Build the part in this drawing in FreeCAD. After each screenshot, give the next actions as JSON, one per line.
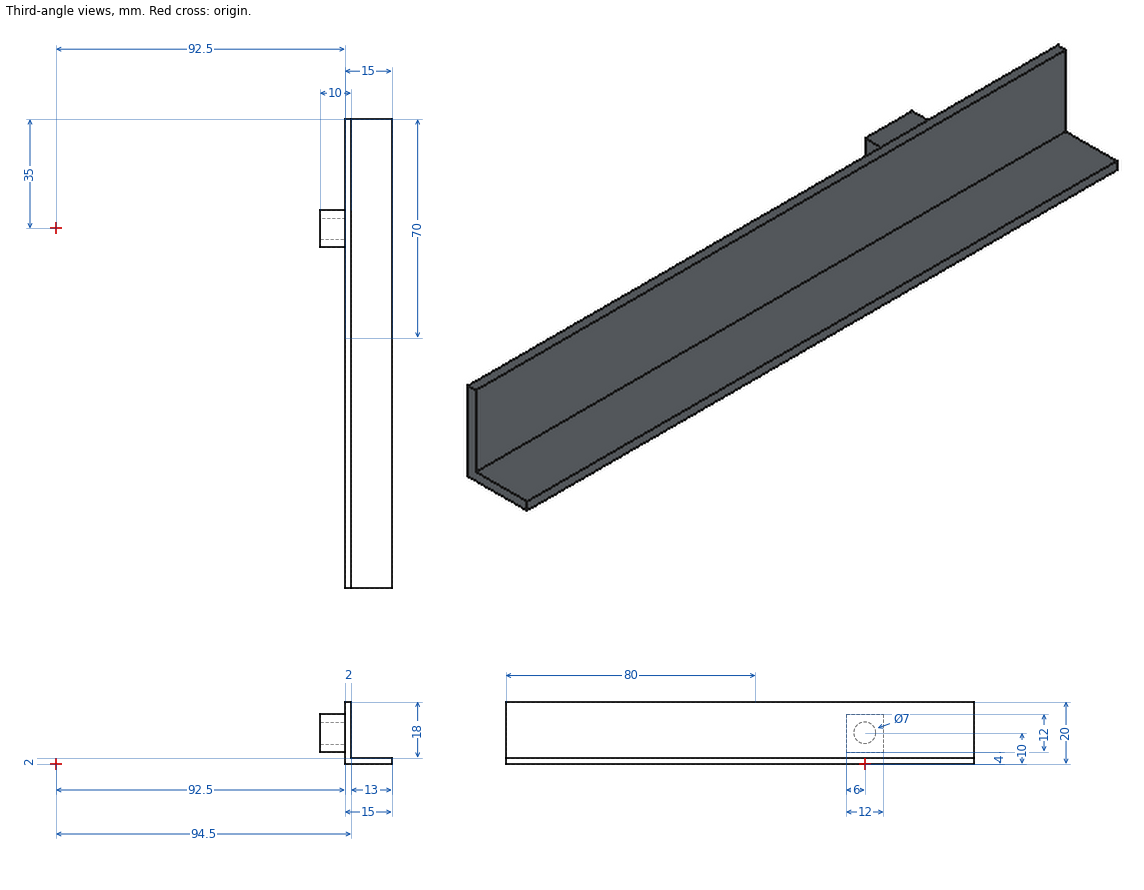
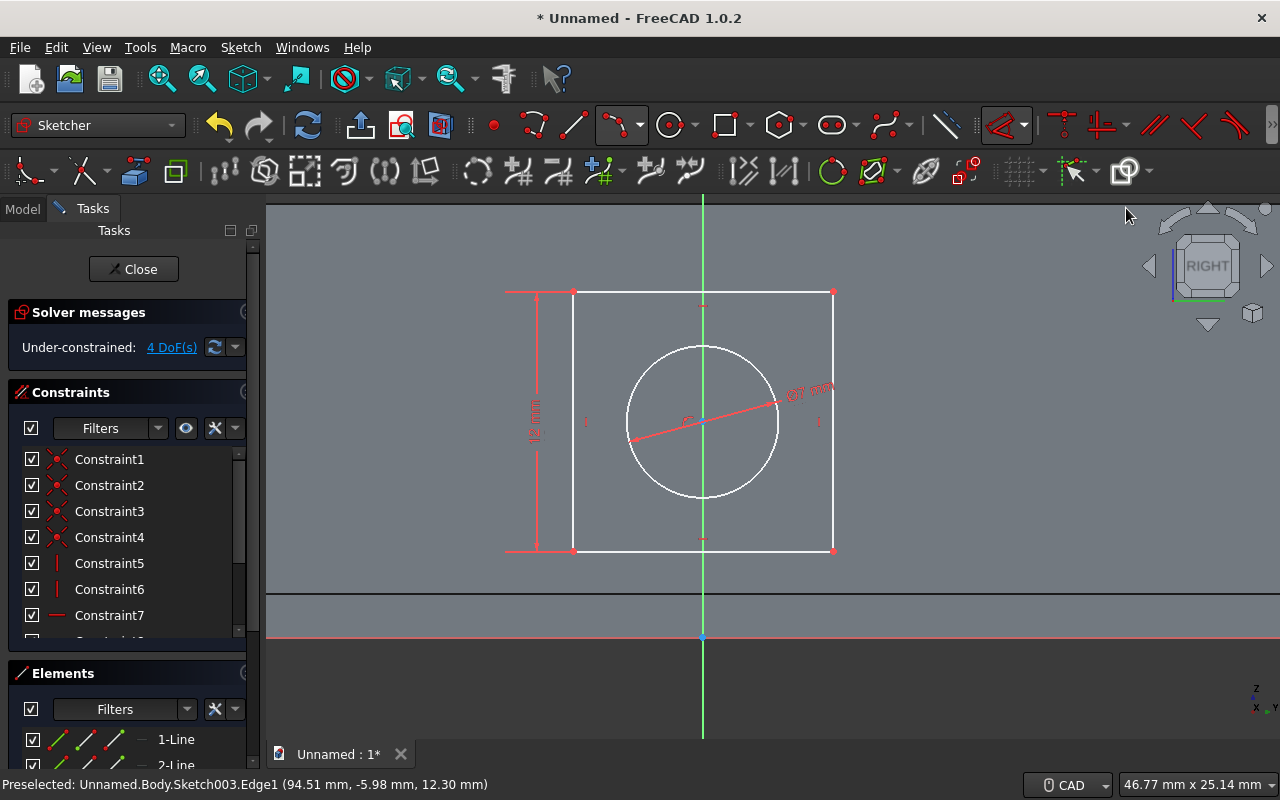
{"action": "left_click", "coordinate": [651, 552]}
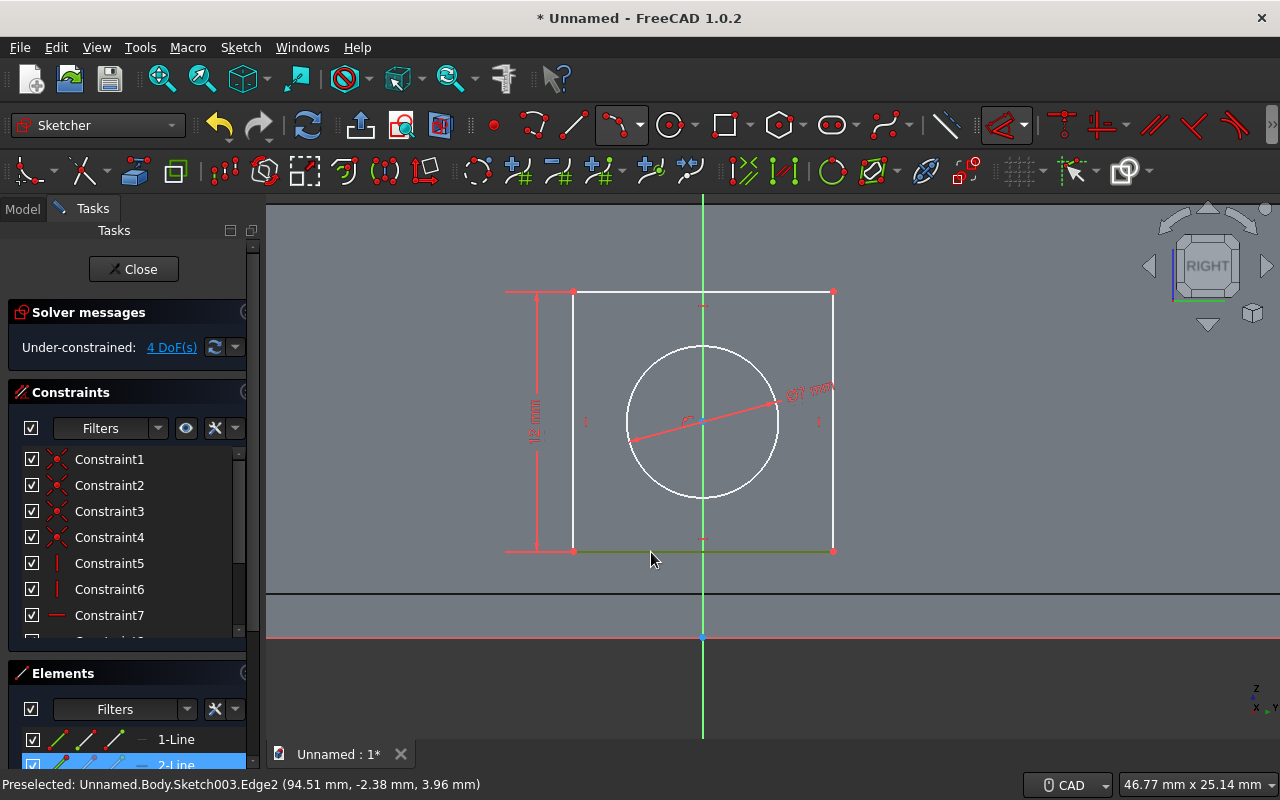
{"action": "key", "text": "l"}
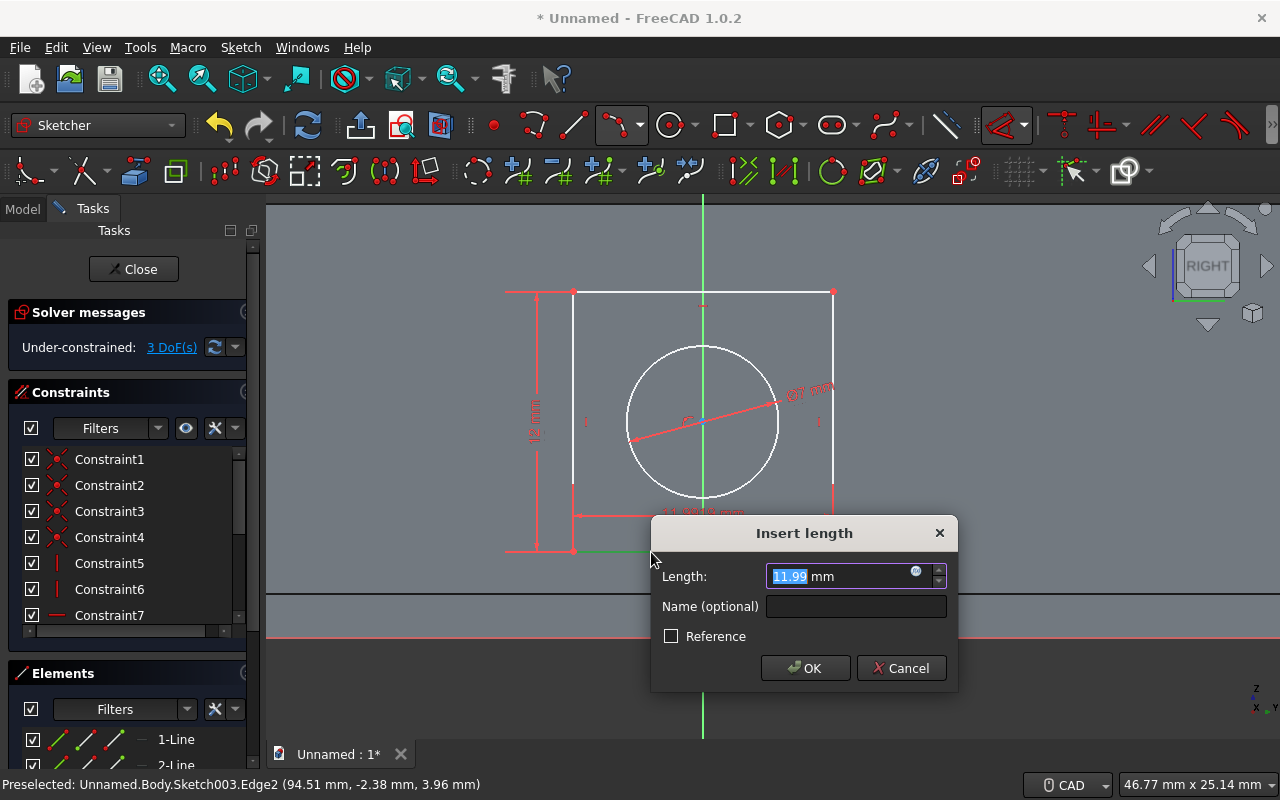
{"action": "type", "text": "12"}
{"action": "key", "text": "Return"}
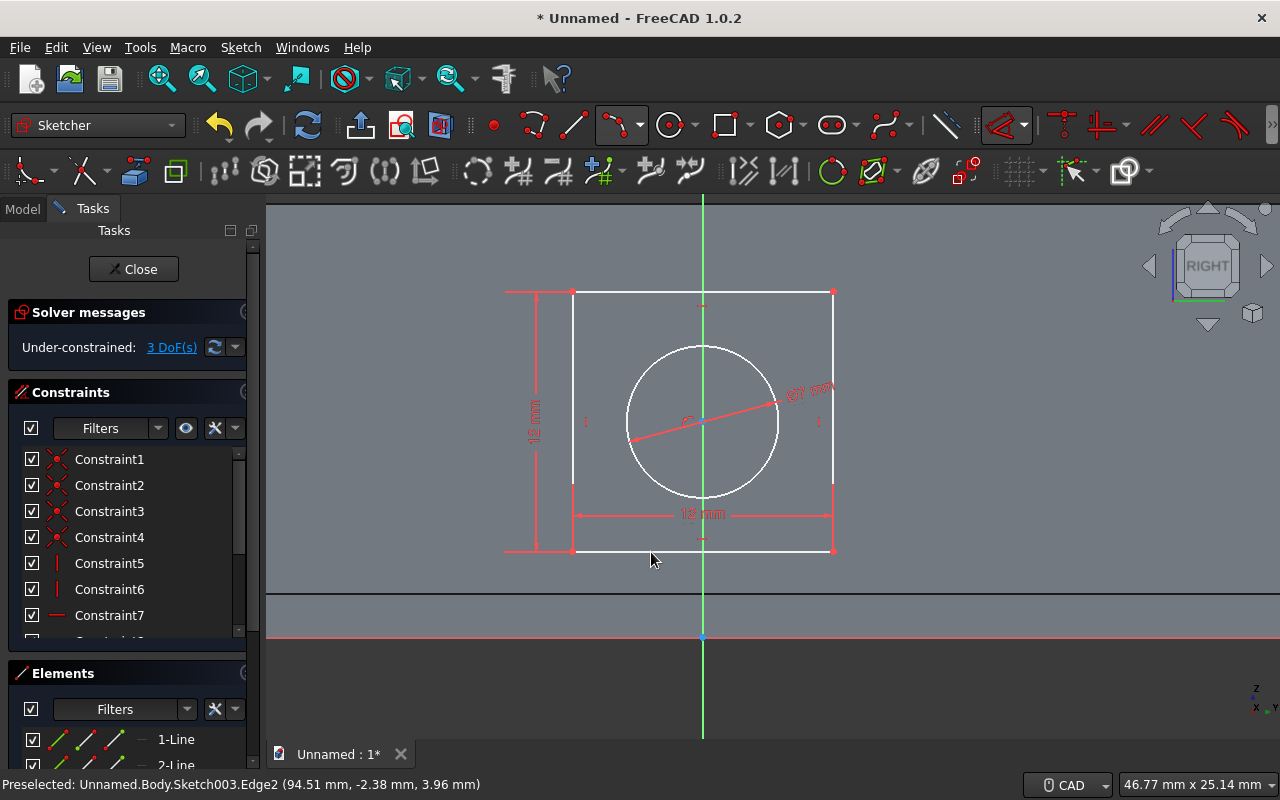
{"action": "left_click", "coordinate": [573, 292]}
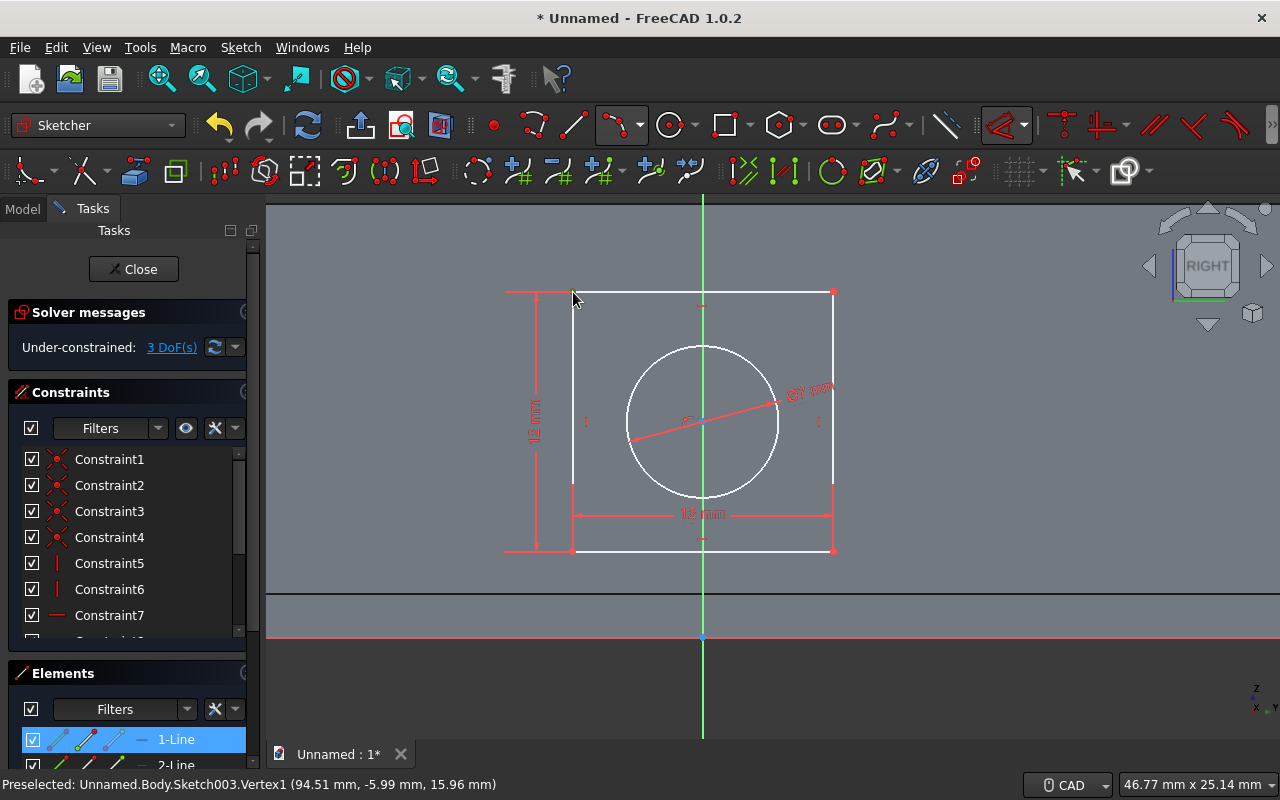
{"action": "left_click", "coordinate": [1026, 126]}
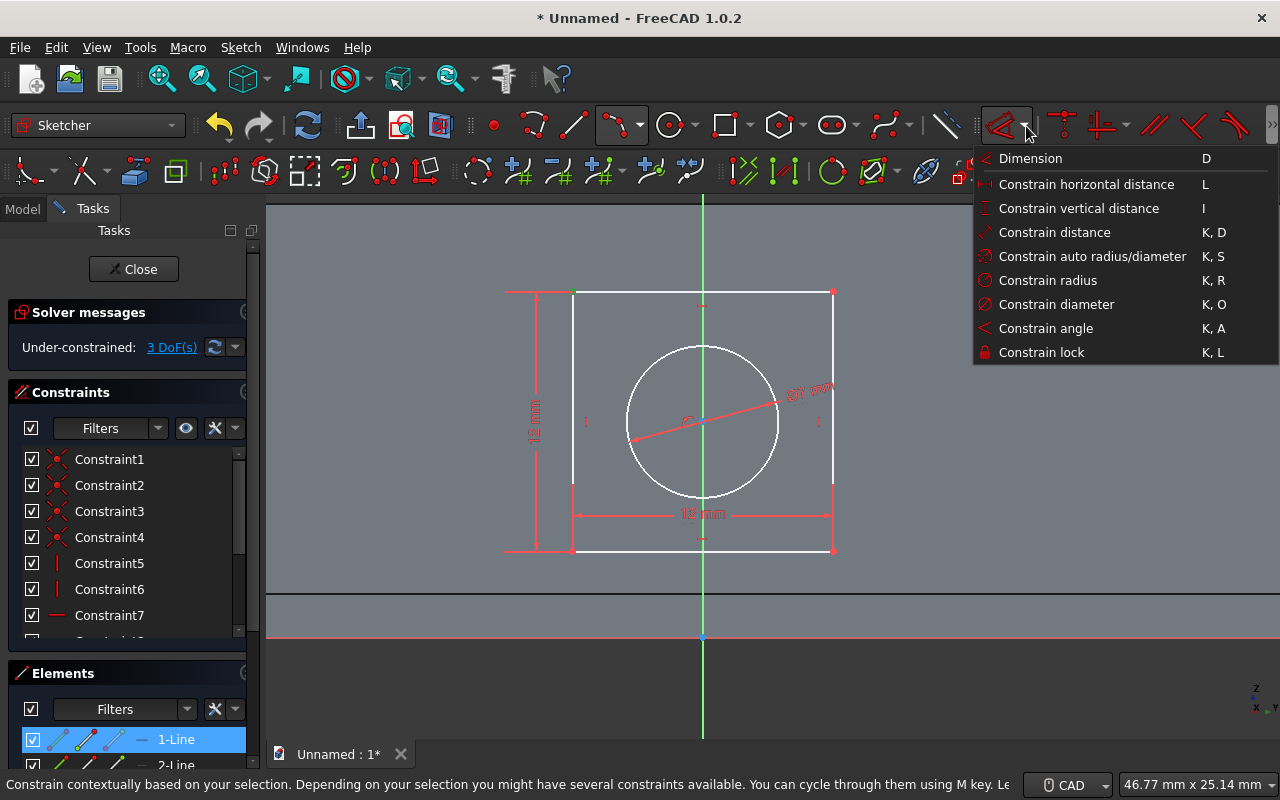
{"action": "left_click", "coordinate": [1126, 184]}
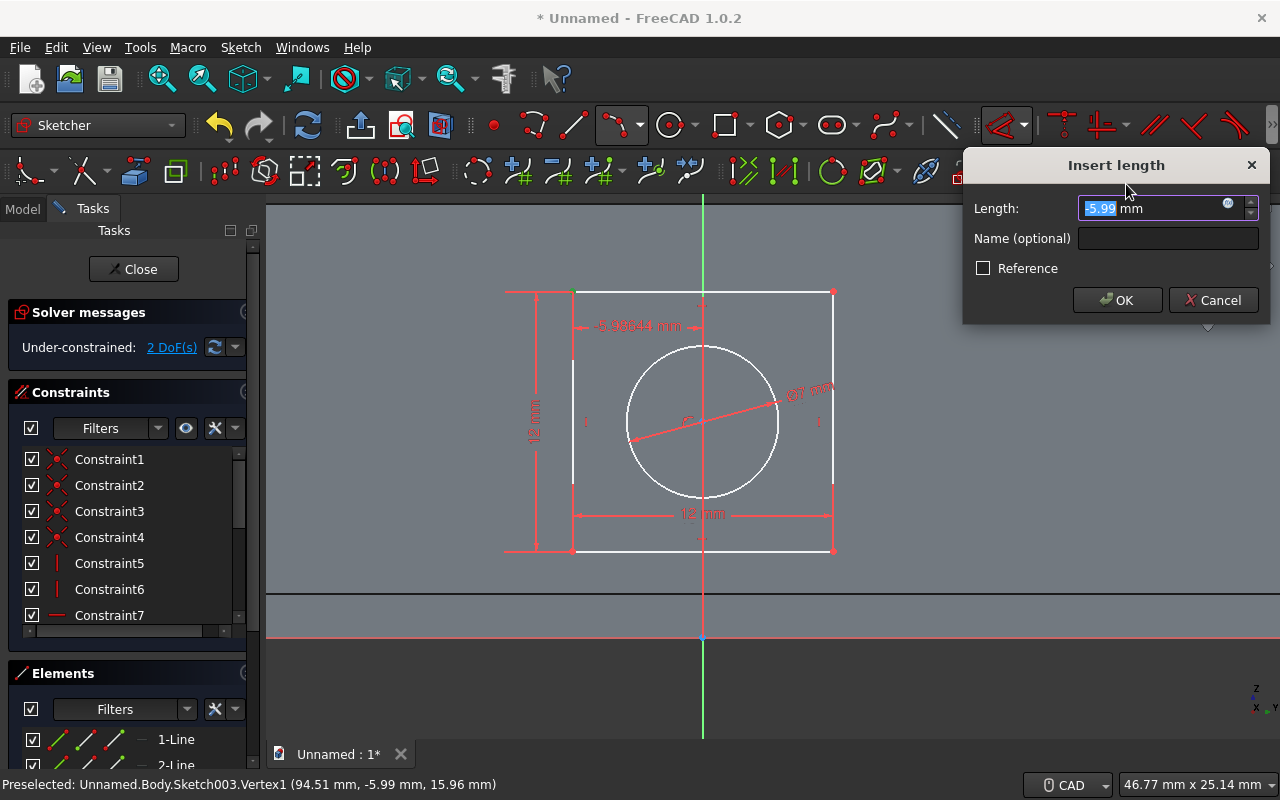
{"action": "type", "text": "-6"}
{"action": "key", "text": "Return"}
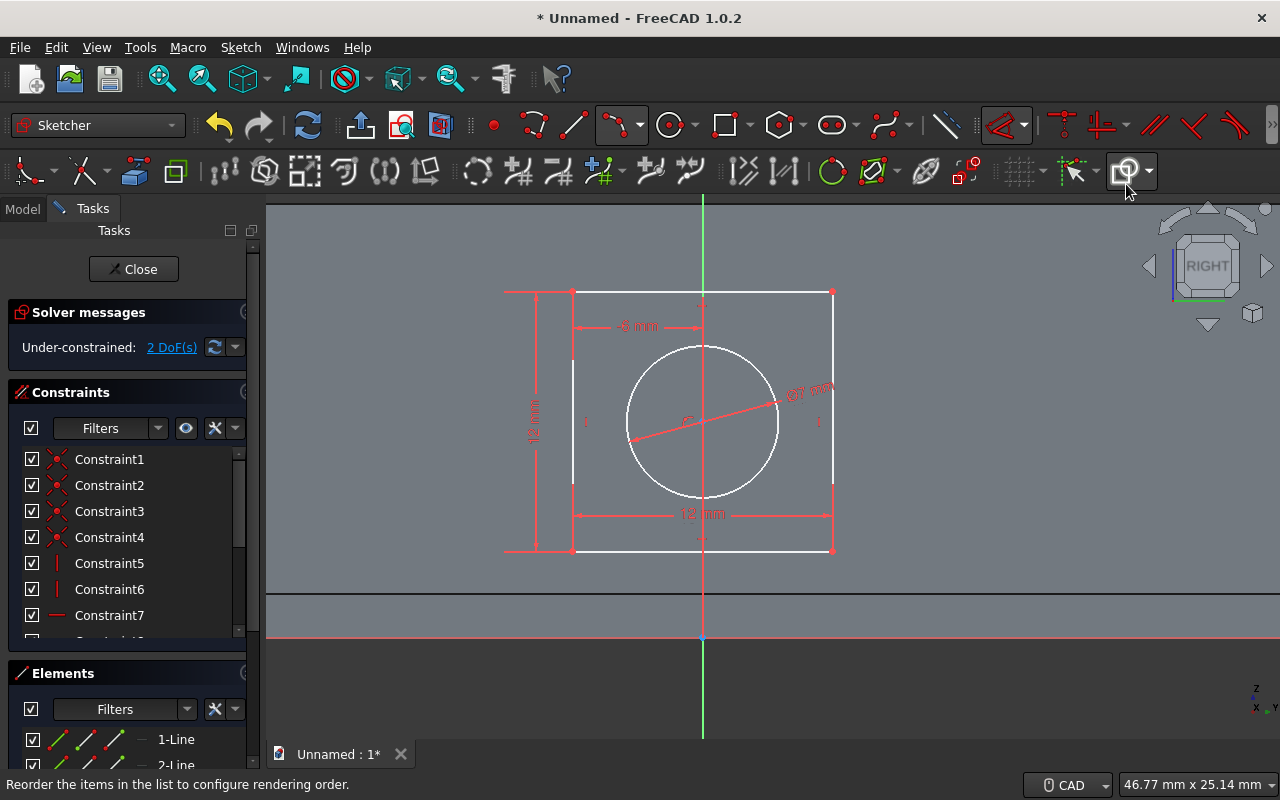
{"action": "left_click", "coordinate": [573, 552]}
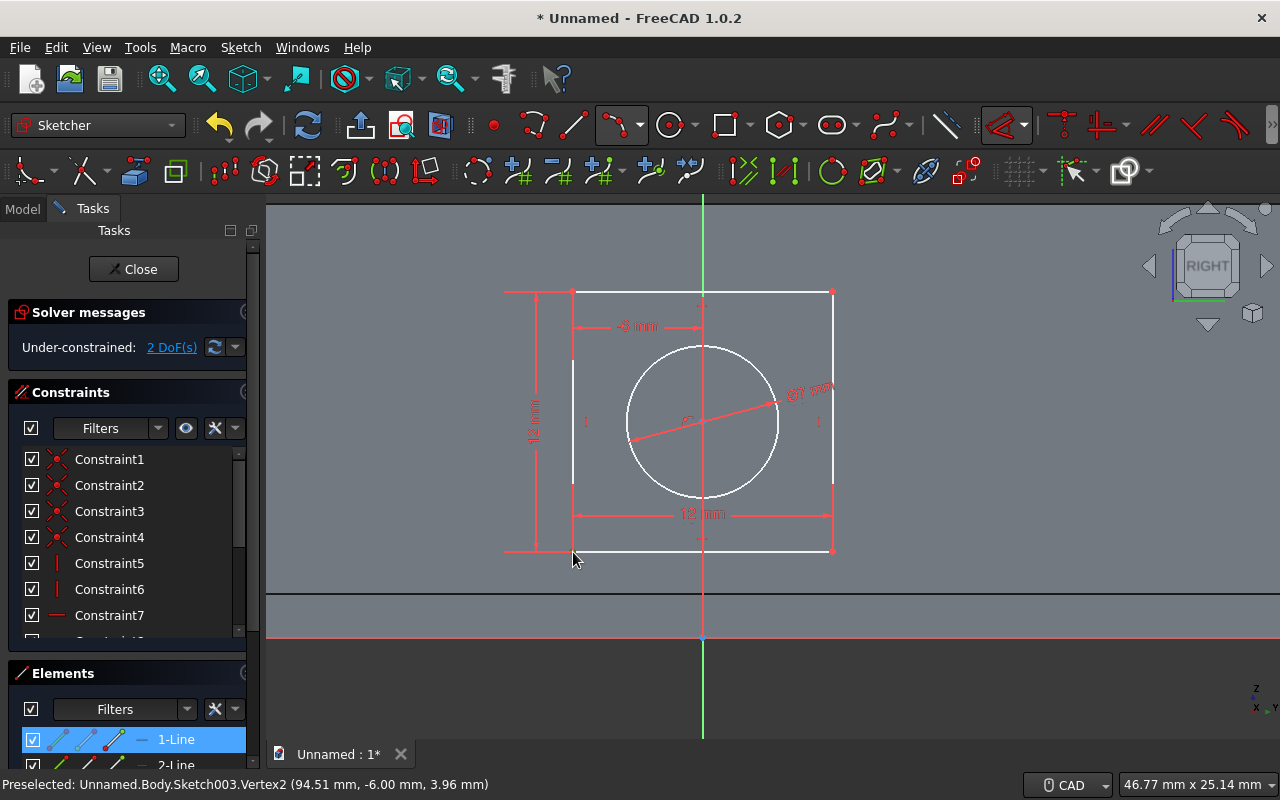
{"action": "key", "text": "i"}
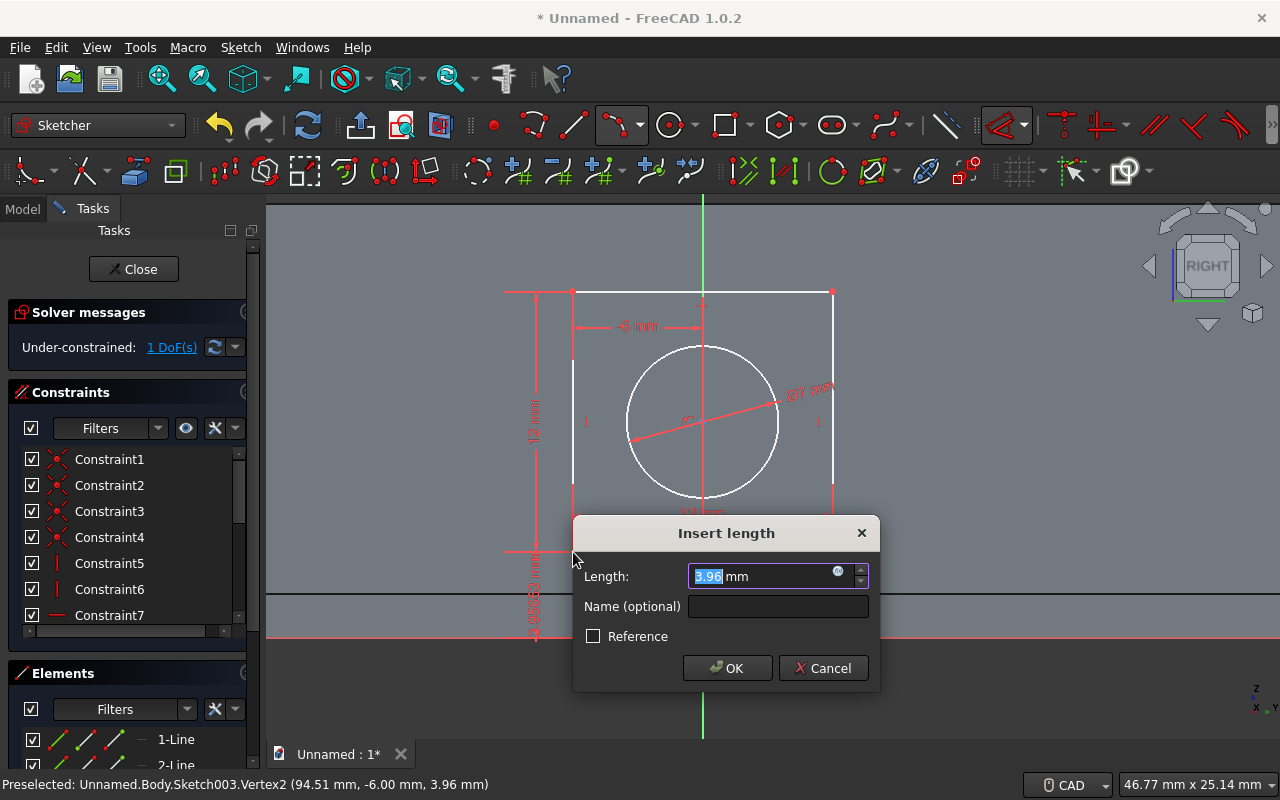
{"action": "type", "text": "4"}
{"action": "key", "text": "Return"}